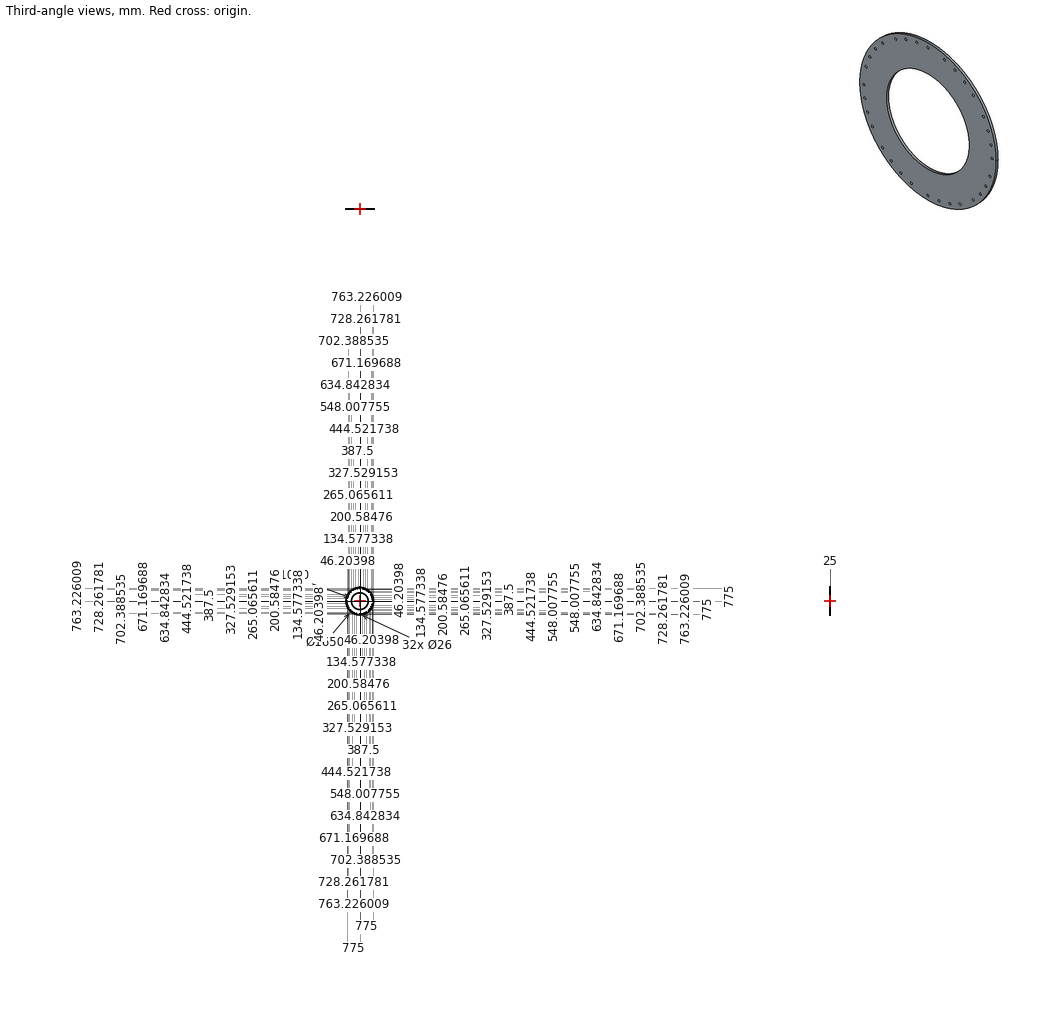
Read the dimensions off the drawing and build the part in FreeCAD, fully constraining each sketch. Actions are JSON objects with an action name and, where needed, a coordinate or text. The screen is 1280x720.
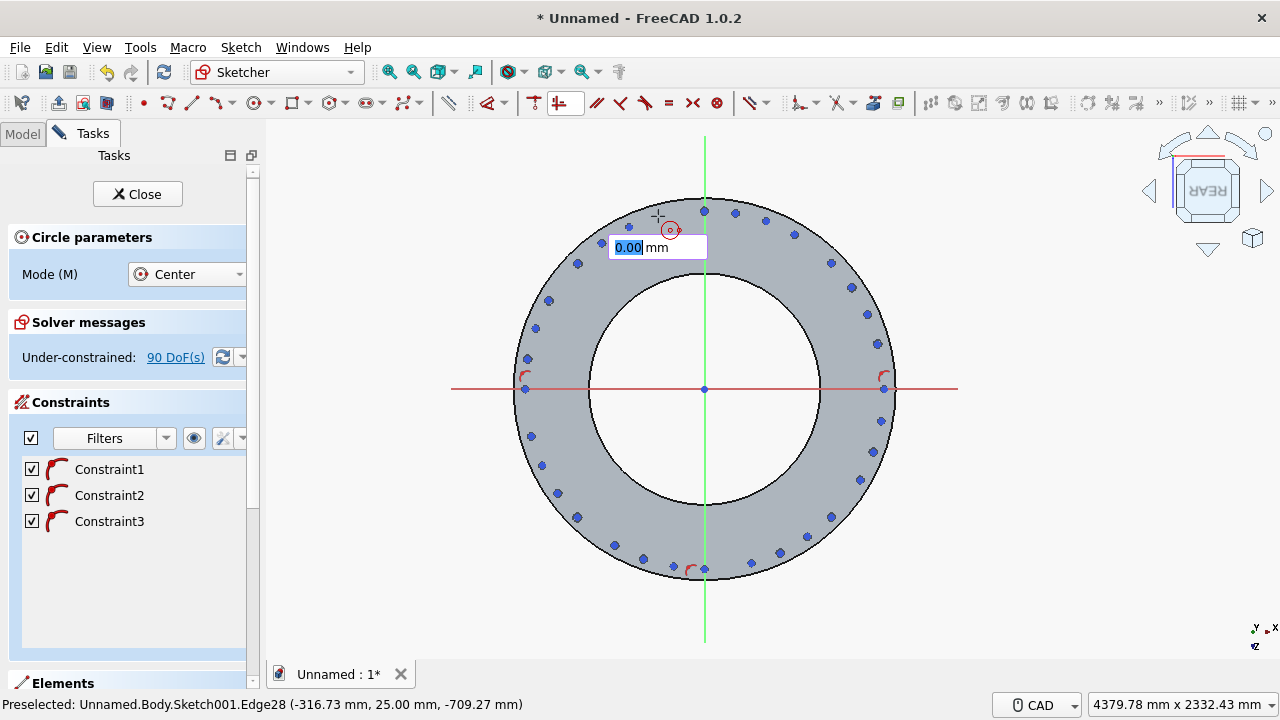
{"action": "scroll", "coordinate": [660, 214], "scroll_direction": "up", "scroll_amount": 9}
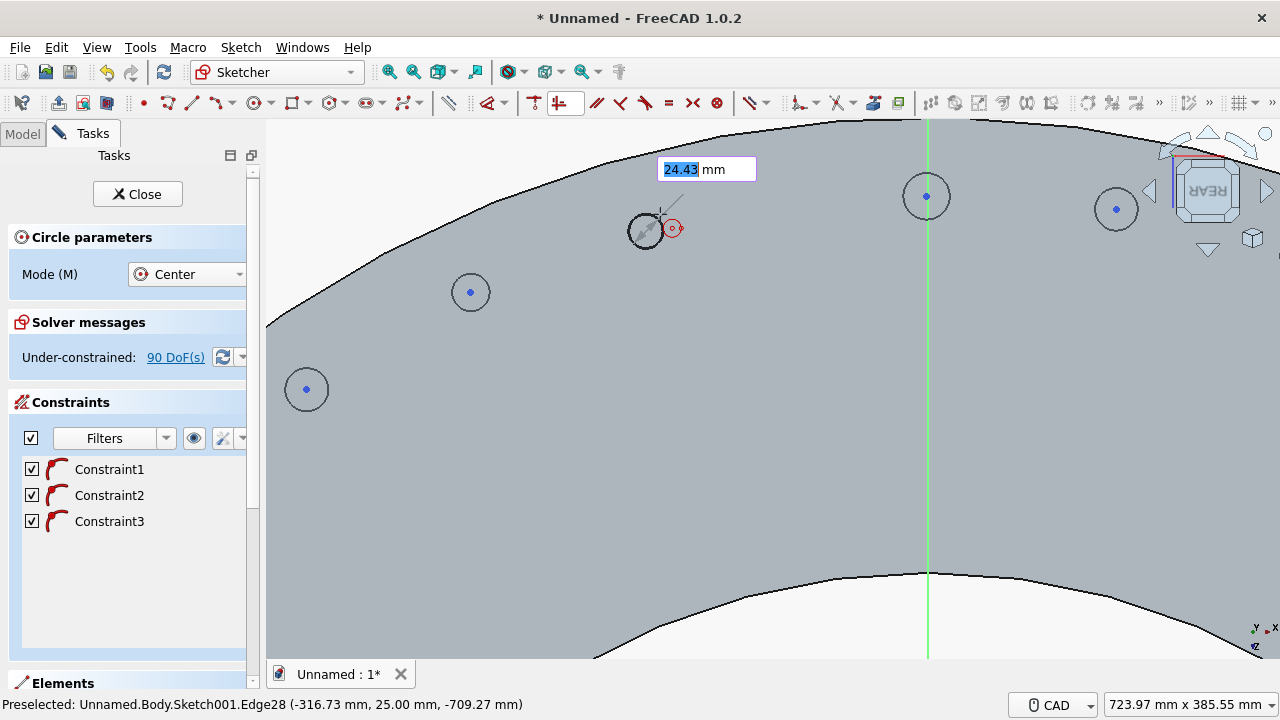
{"action": "left_click", "coordinate": [660, 212]}
{"action": "key", "text": "Escape"}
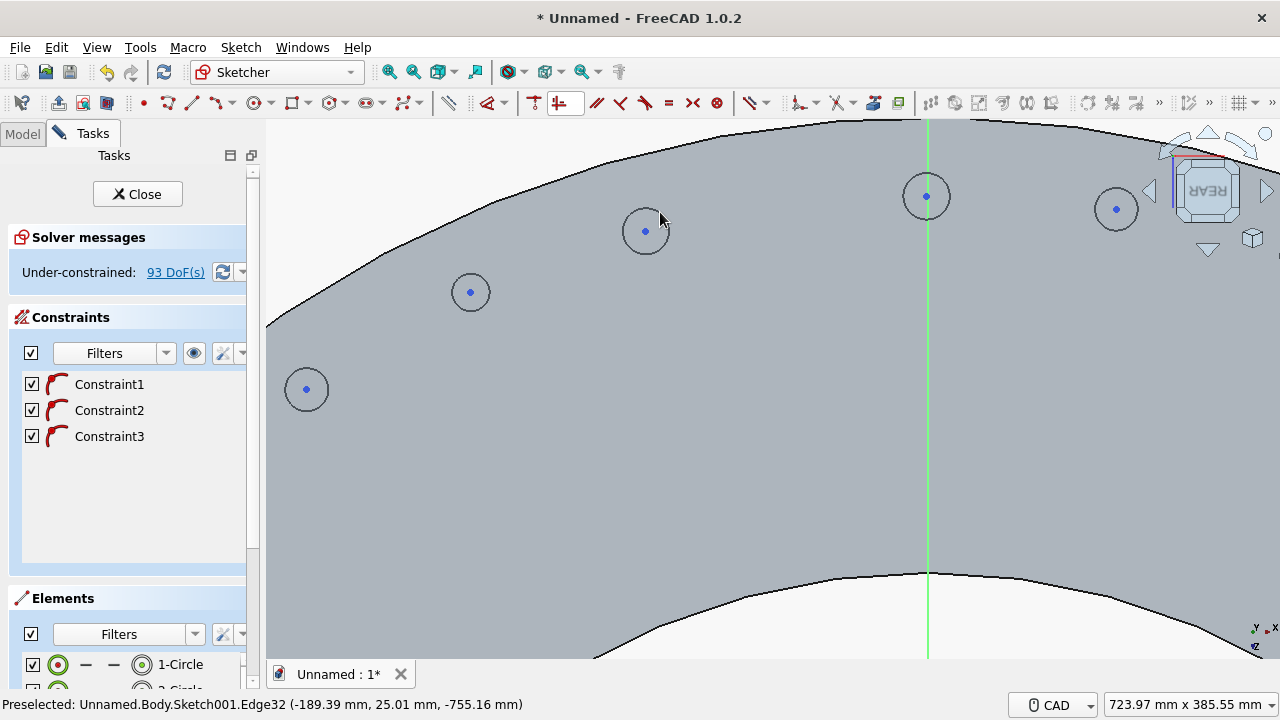
{"action": "left_click", "coordinate": [943, 180]}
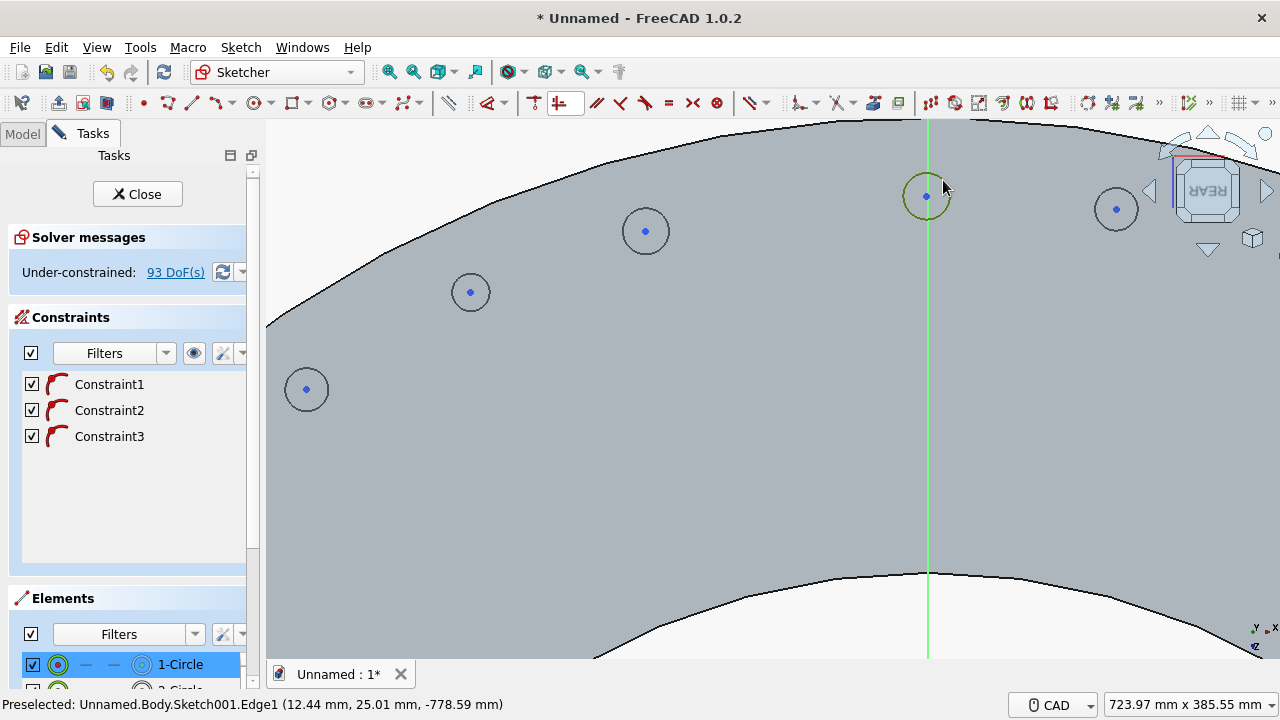
{"action": "left_click", "coordinate": [1101, 194]}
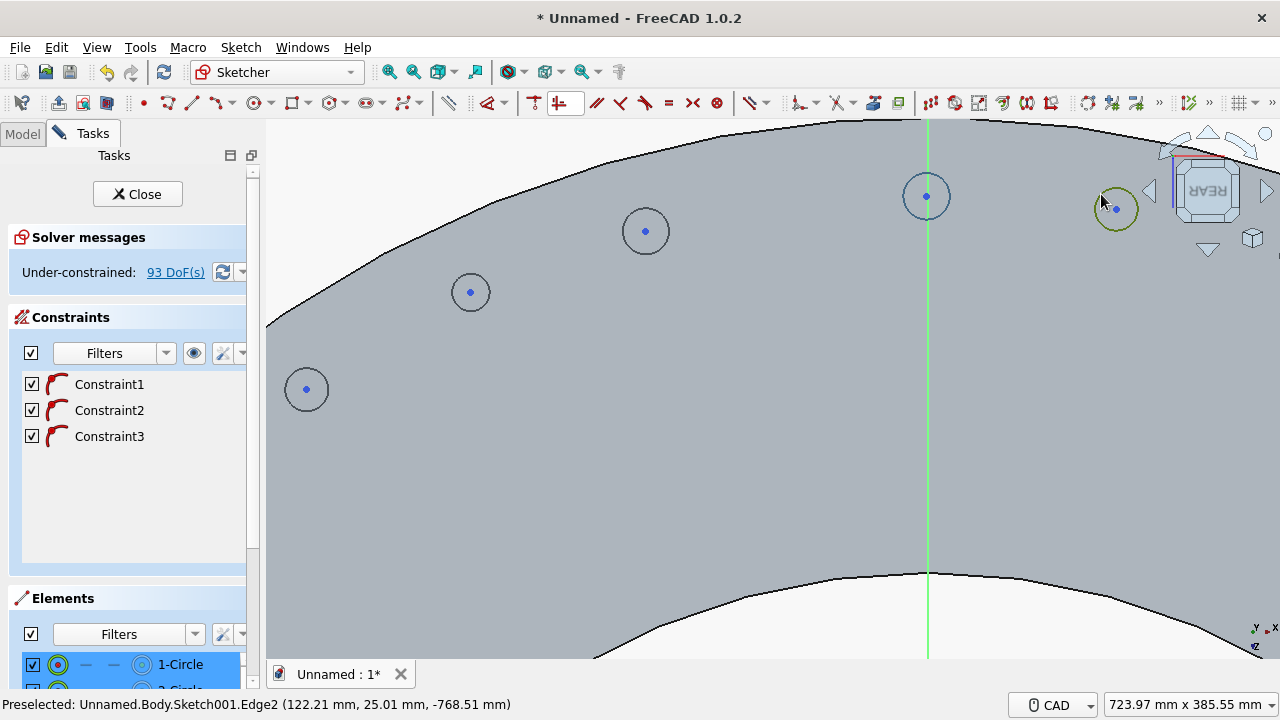
{"action": "scroll", "coordinate": [660, 214], "scroll_direction": "down", "scroll_amount": 9}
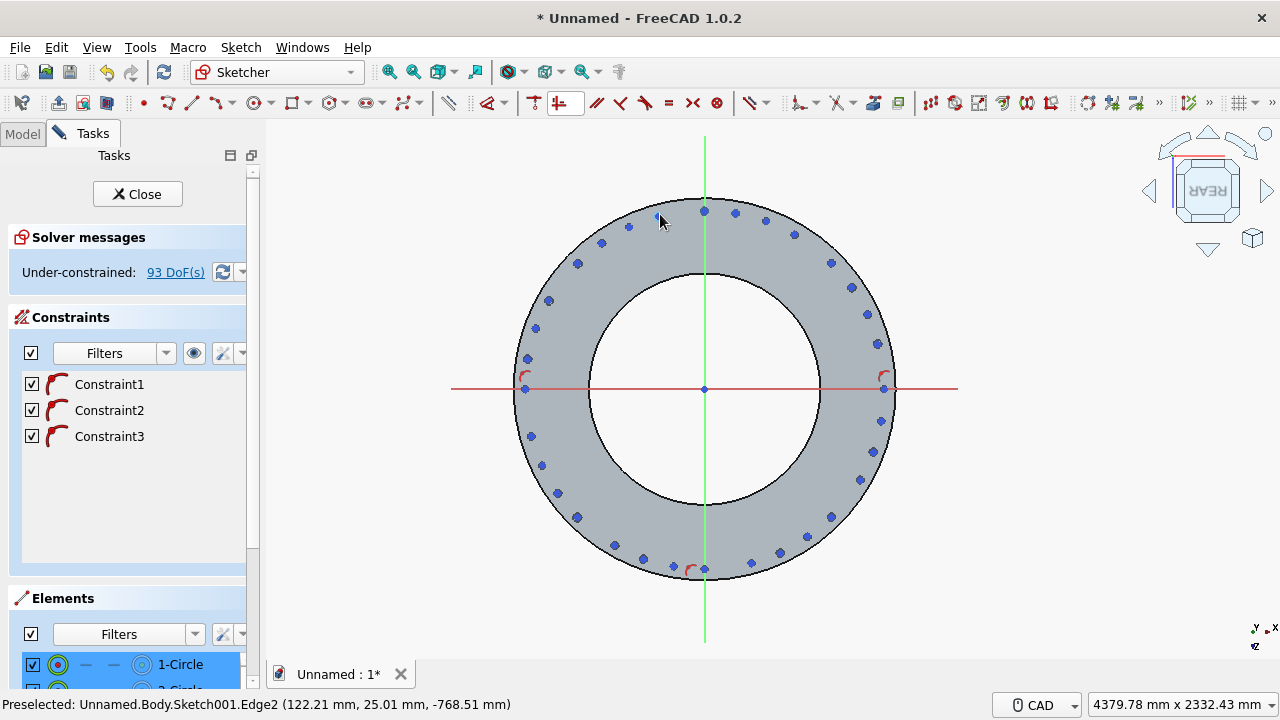
{"action": "scroll", "coordinate": [768, 219], "scroll_direction": "up", "scroll_amount": 8}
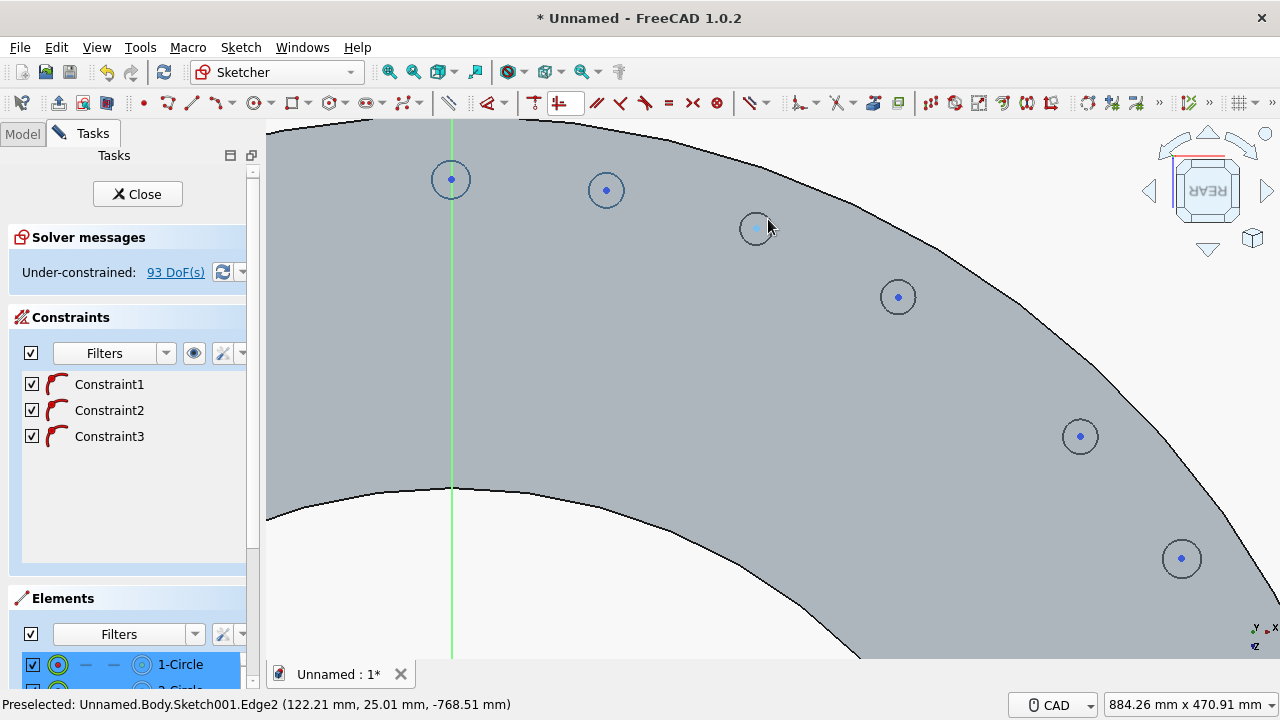
{"action": "left_click", "coordinate": [768, 217]}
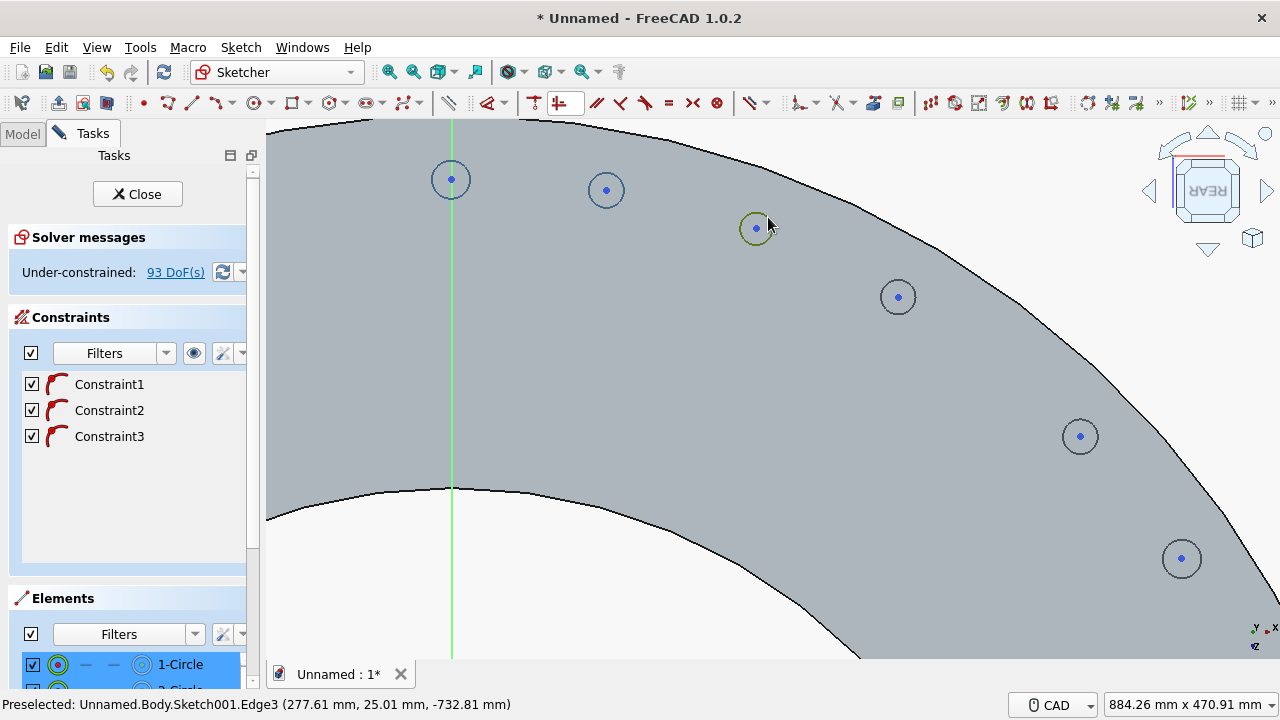
{"action": "left_click", "coordinate": [910, 285]}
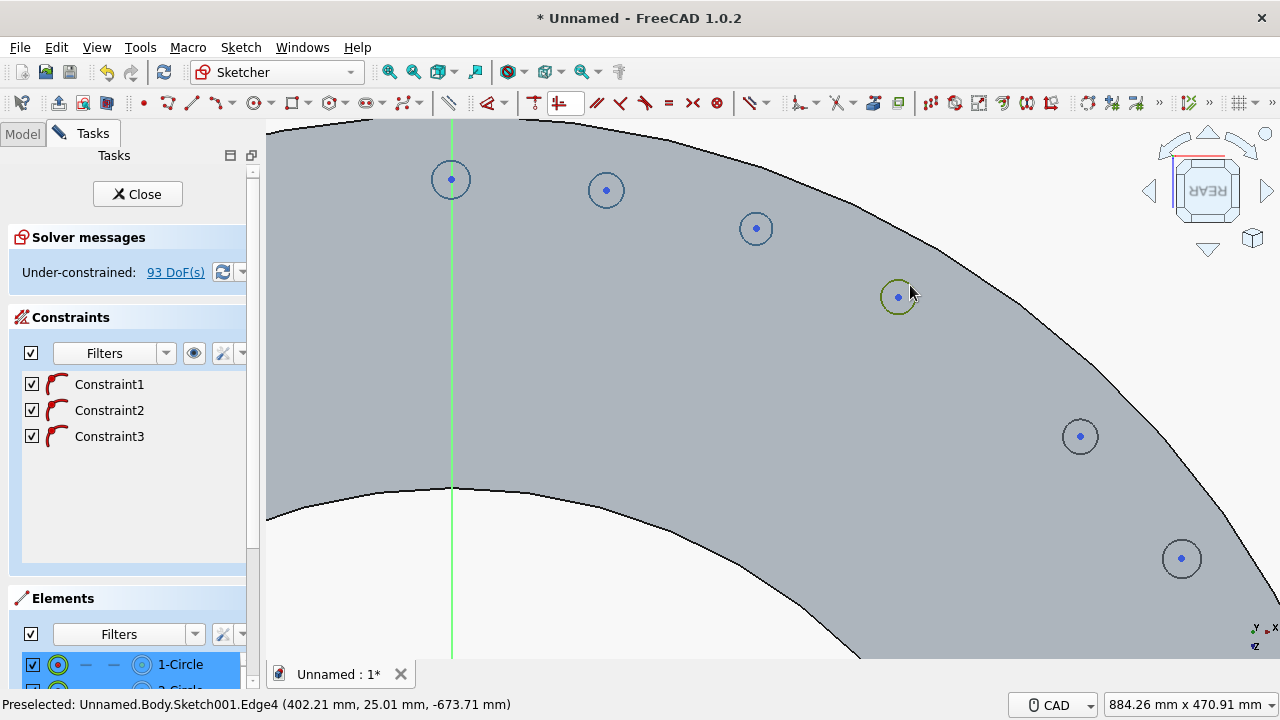
{"action": "left_click", "coordinate": [1093, 424]}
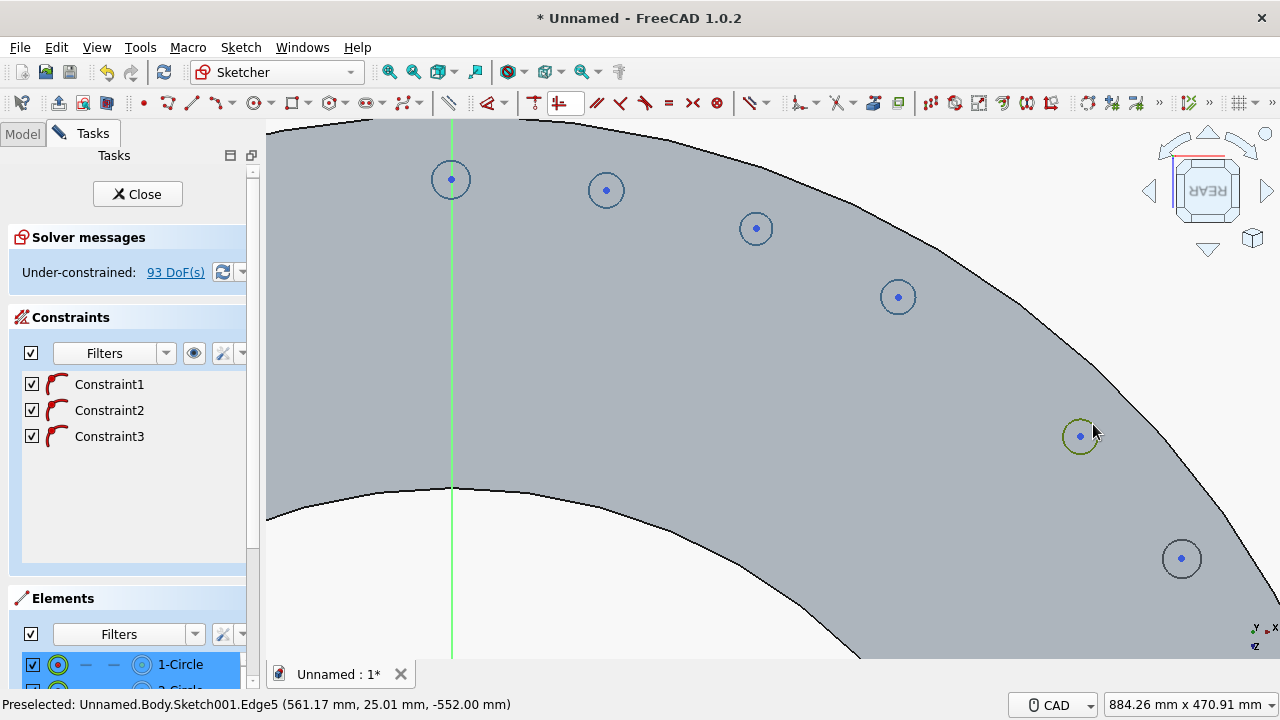
{"action": "scroll", "coordinate": [768, 219], "scroll_direction": "down", "scroll_amount": 8}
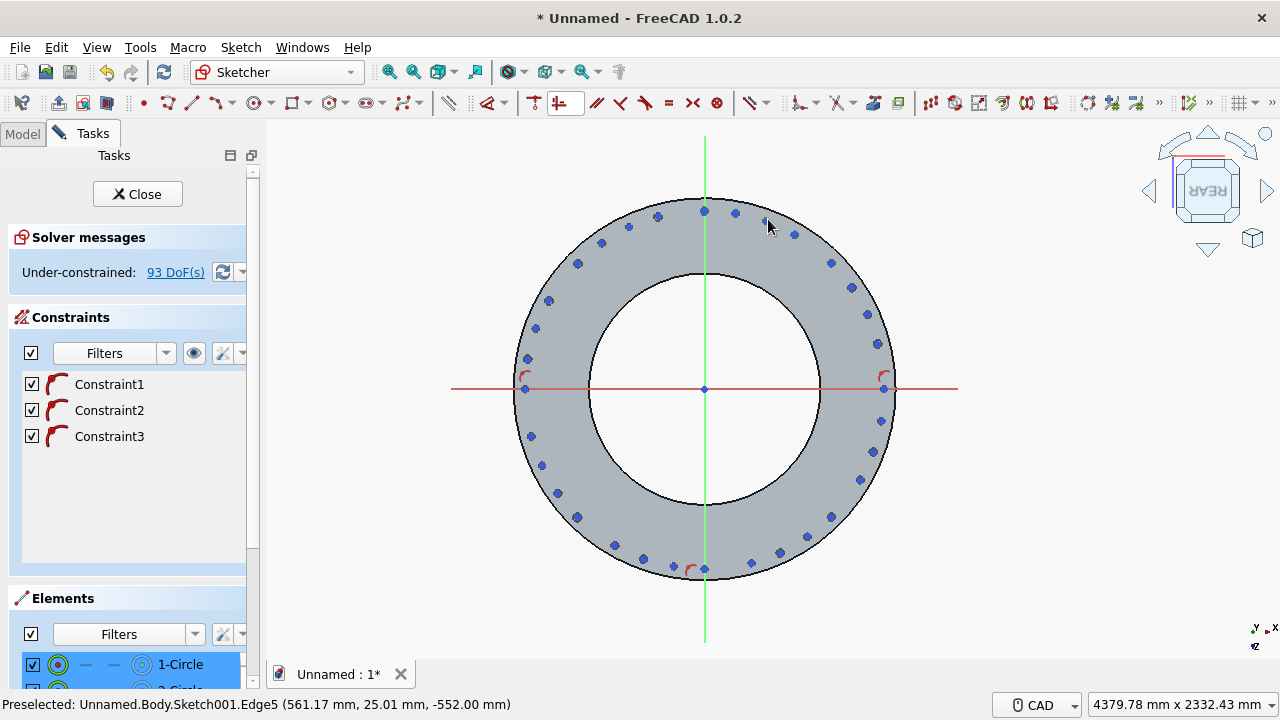
{"action": "scroll", "coordinate": [855, 285], "scroll_direction": "up", "scroll_amount": 7}